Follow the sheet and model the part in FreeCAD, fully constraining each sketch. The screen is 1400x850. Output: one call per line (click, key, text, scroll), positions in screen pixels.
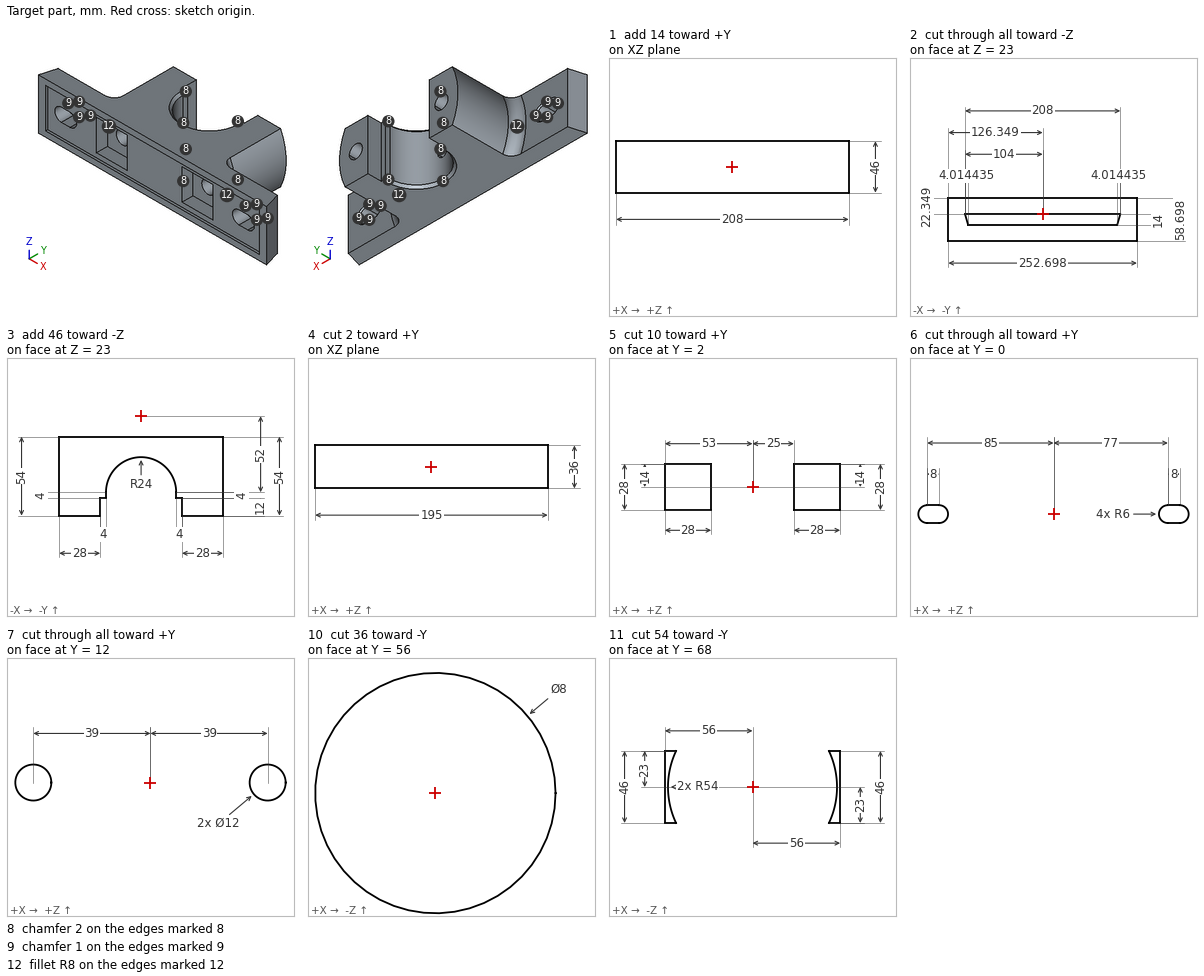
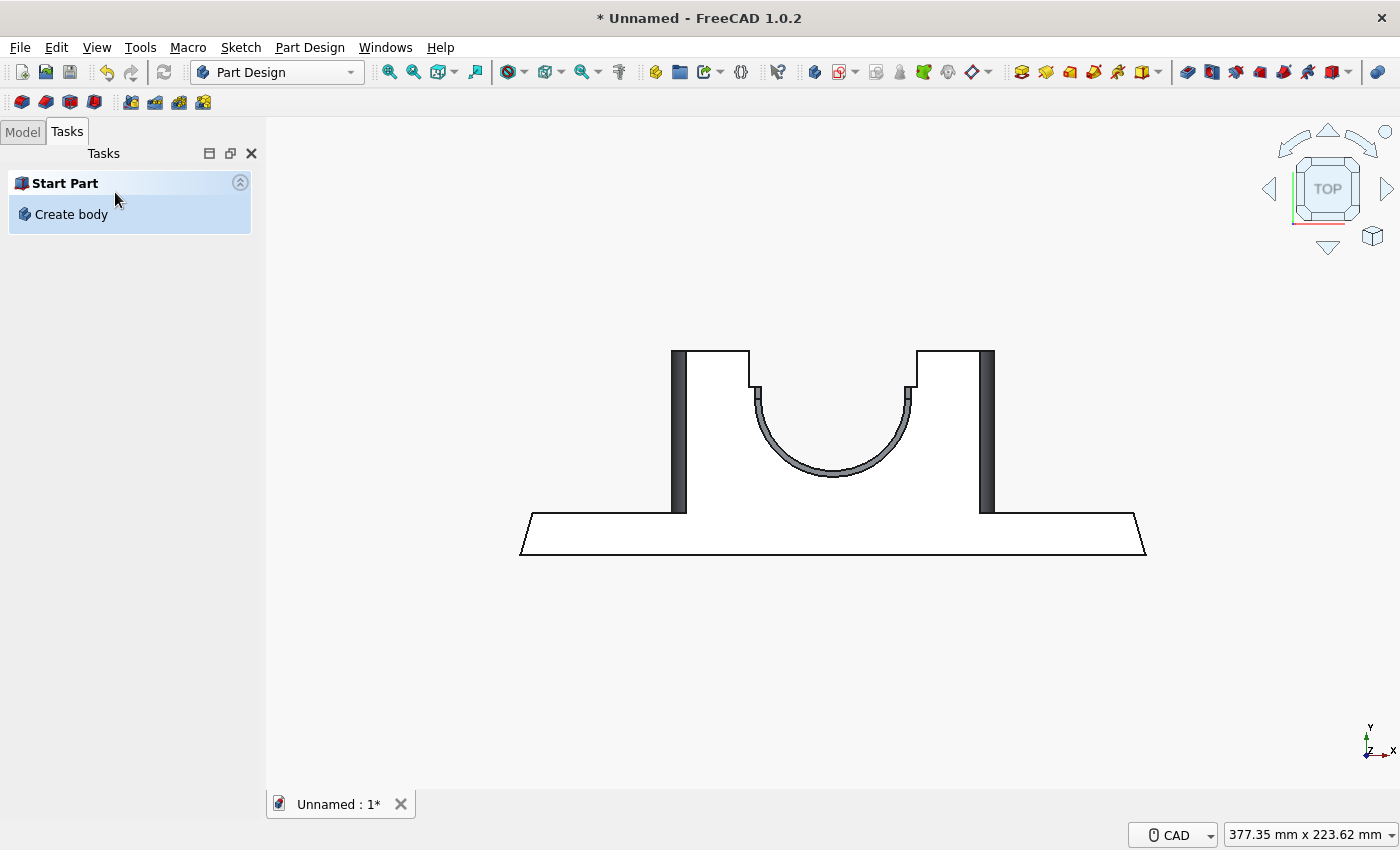
key(1)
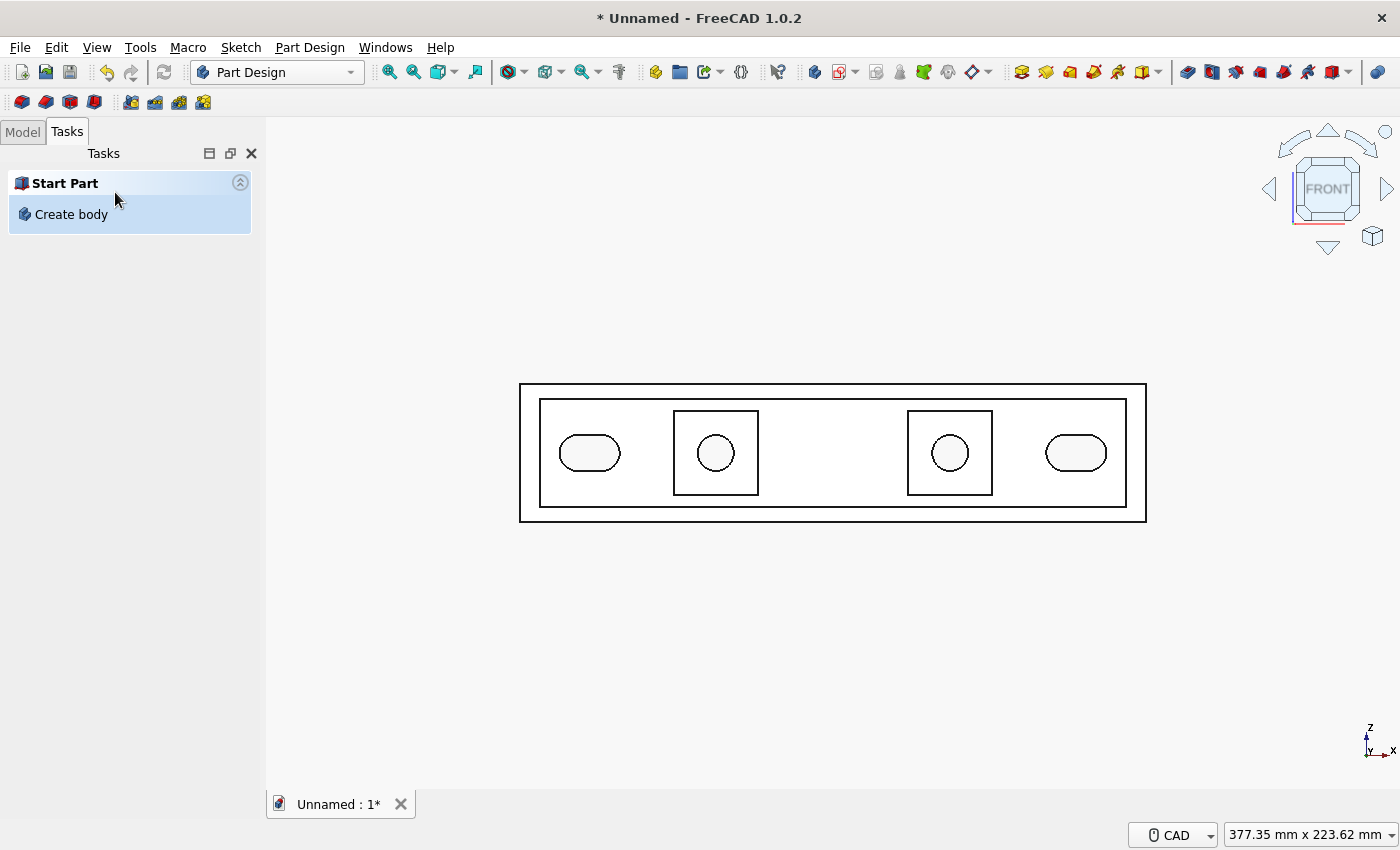
key(3)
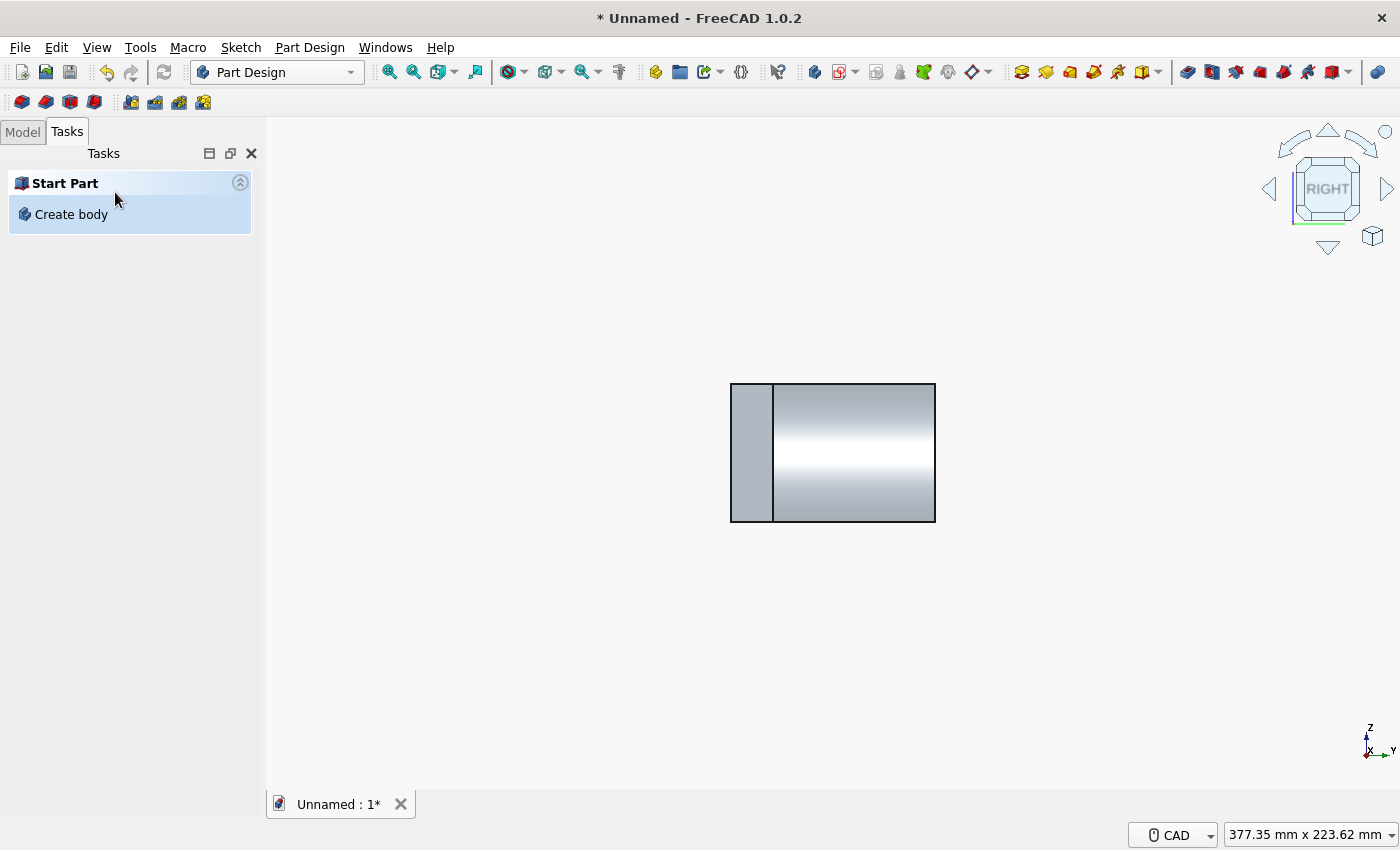
key(v)
key(f)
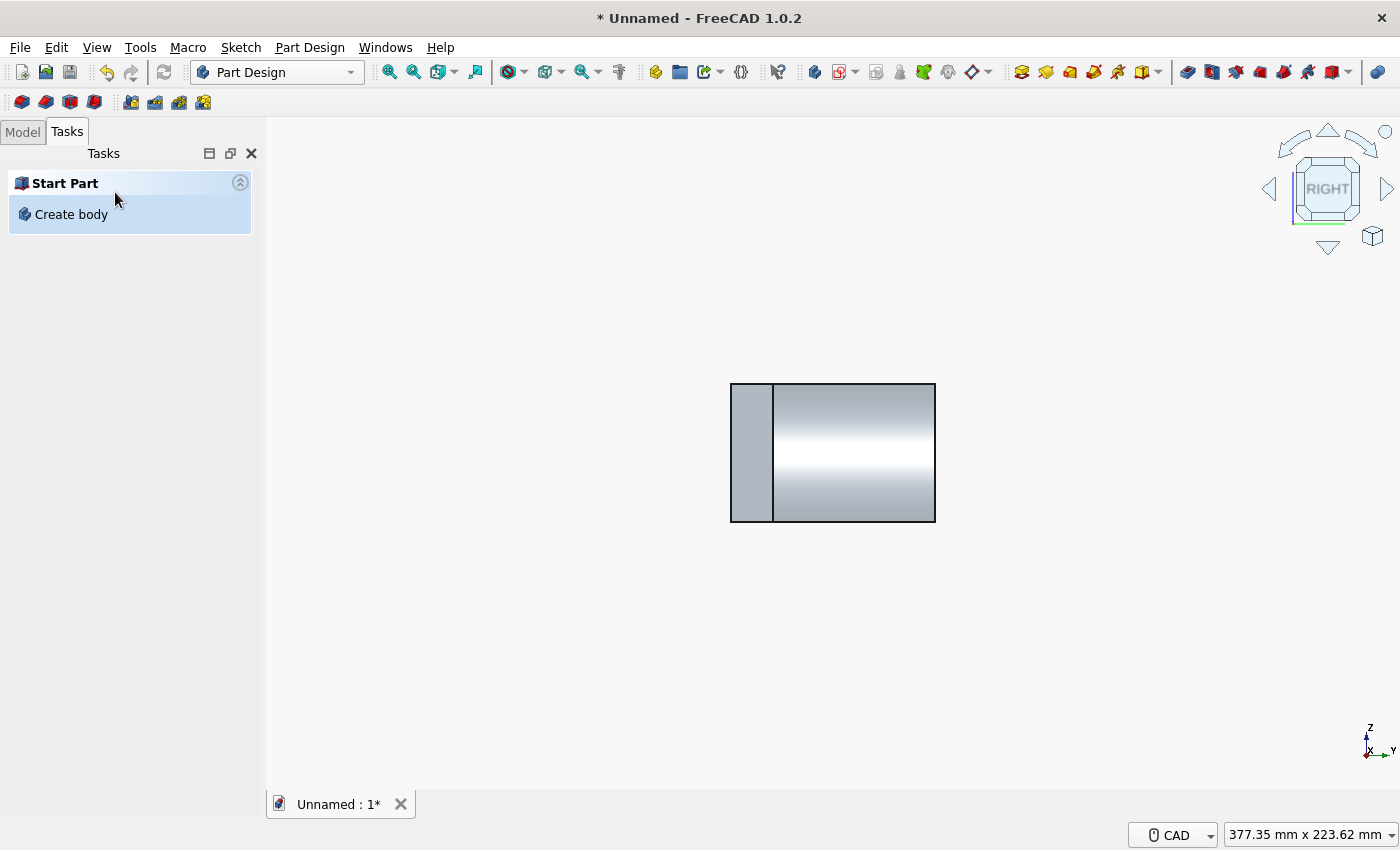
key(5)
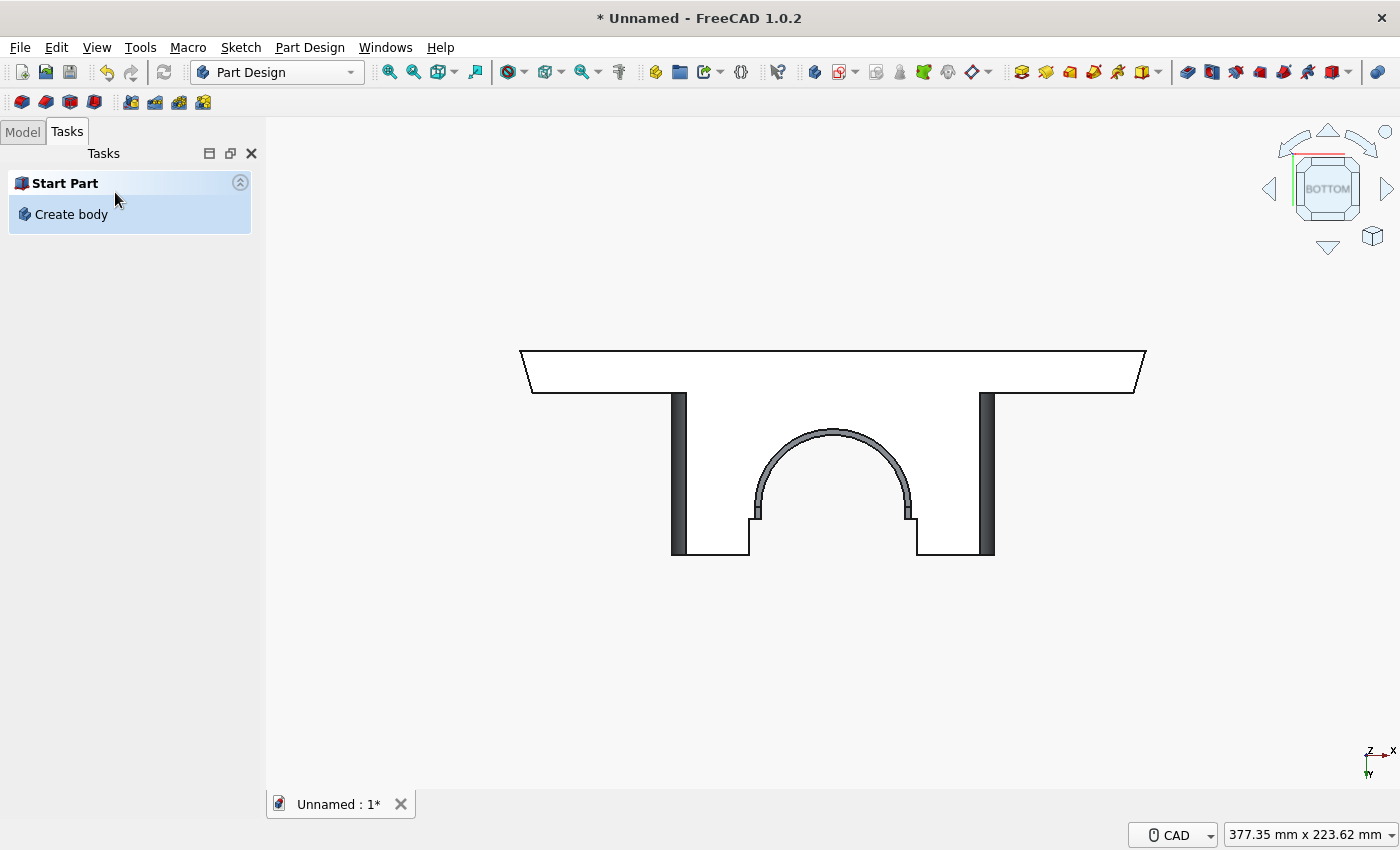
key(4)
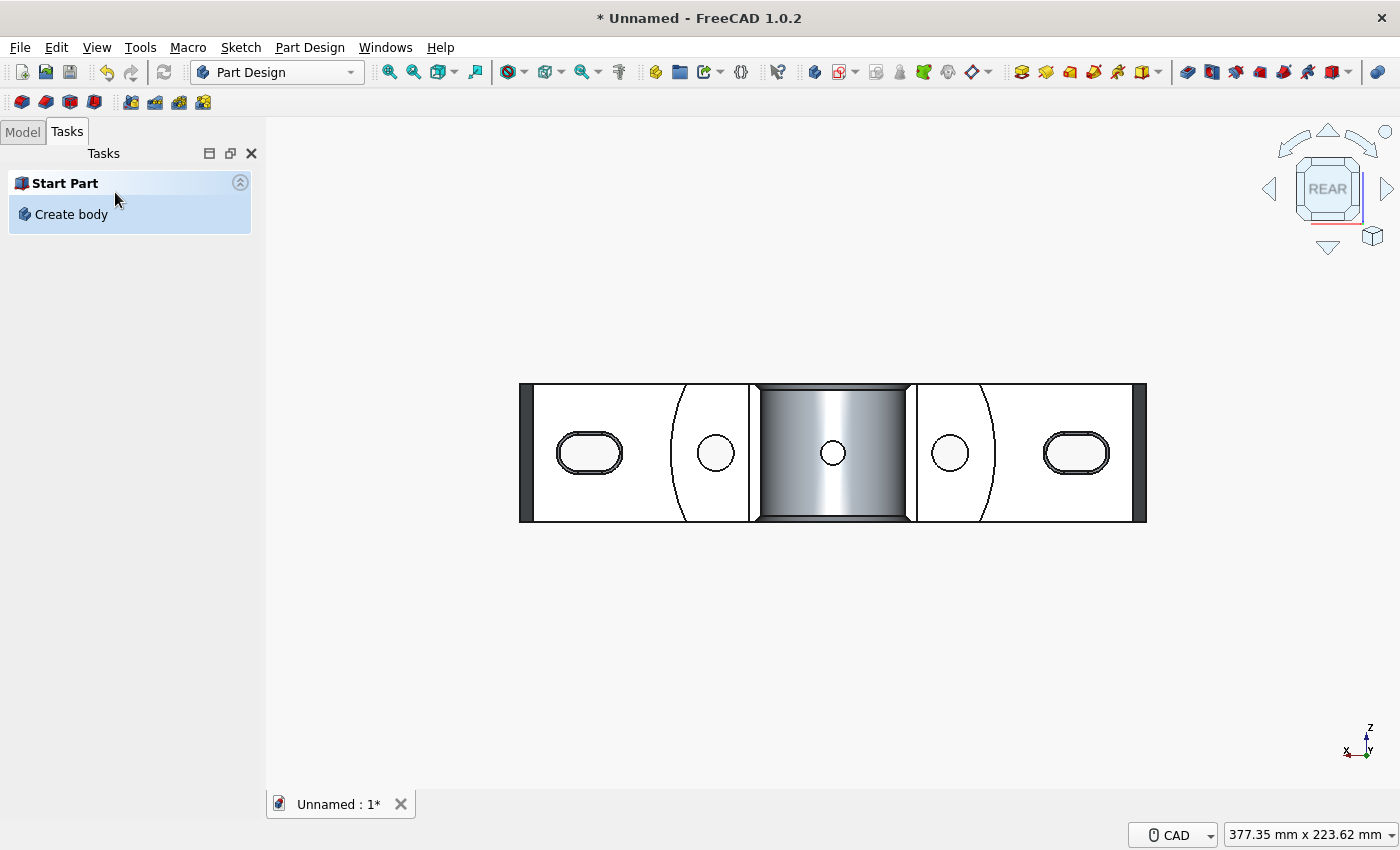
key(6)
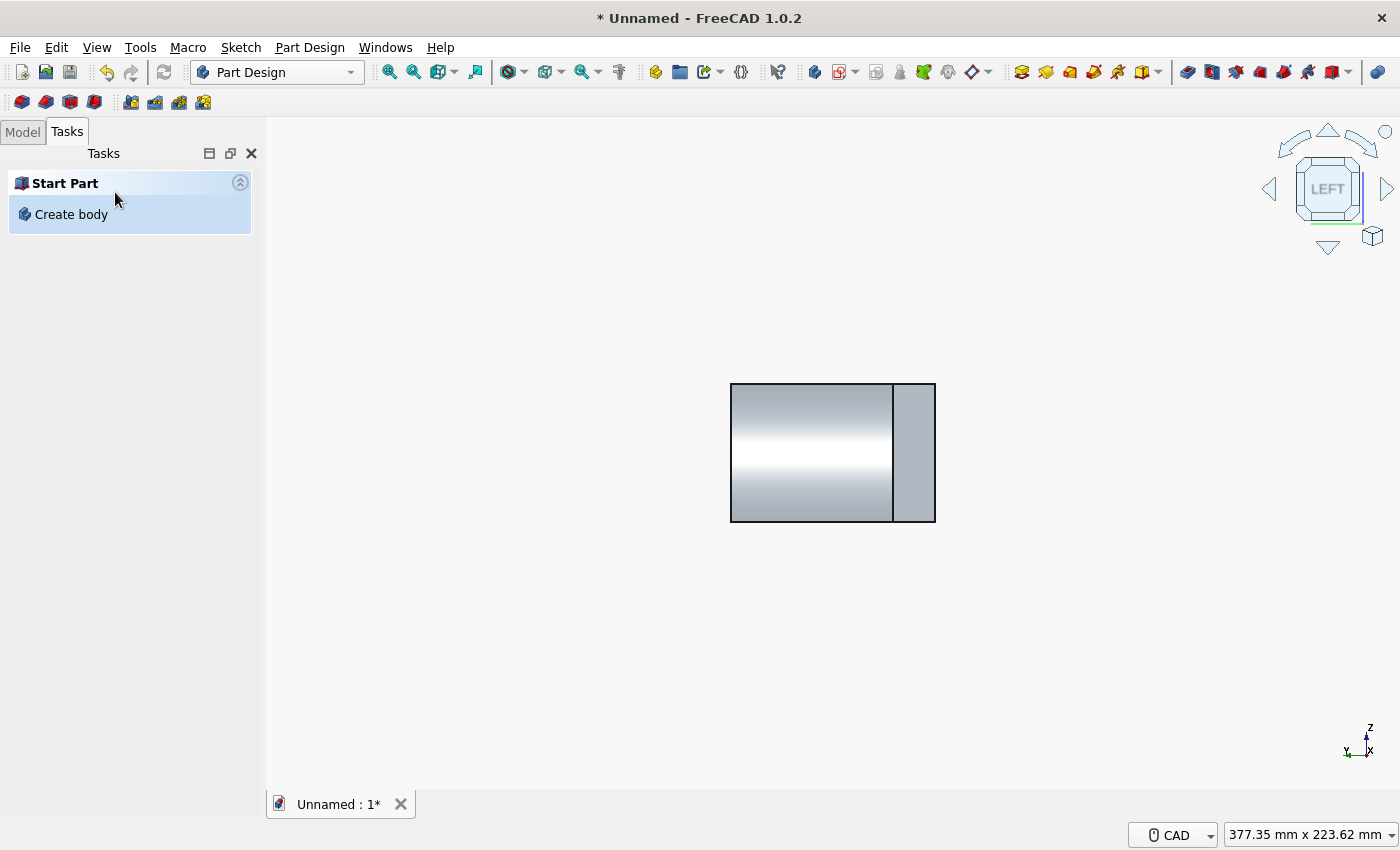
key(v)
key(f)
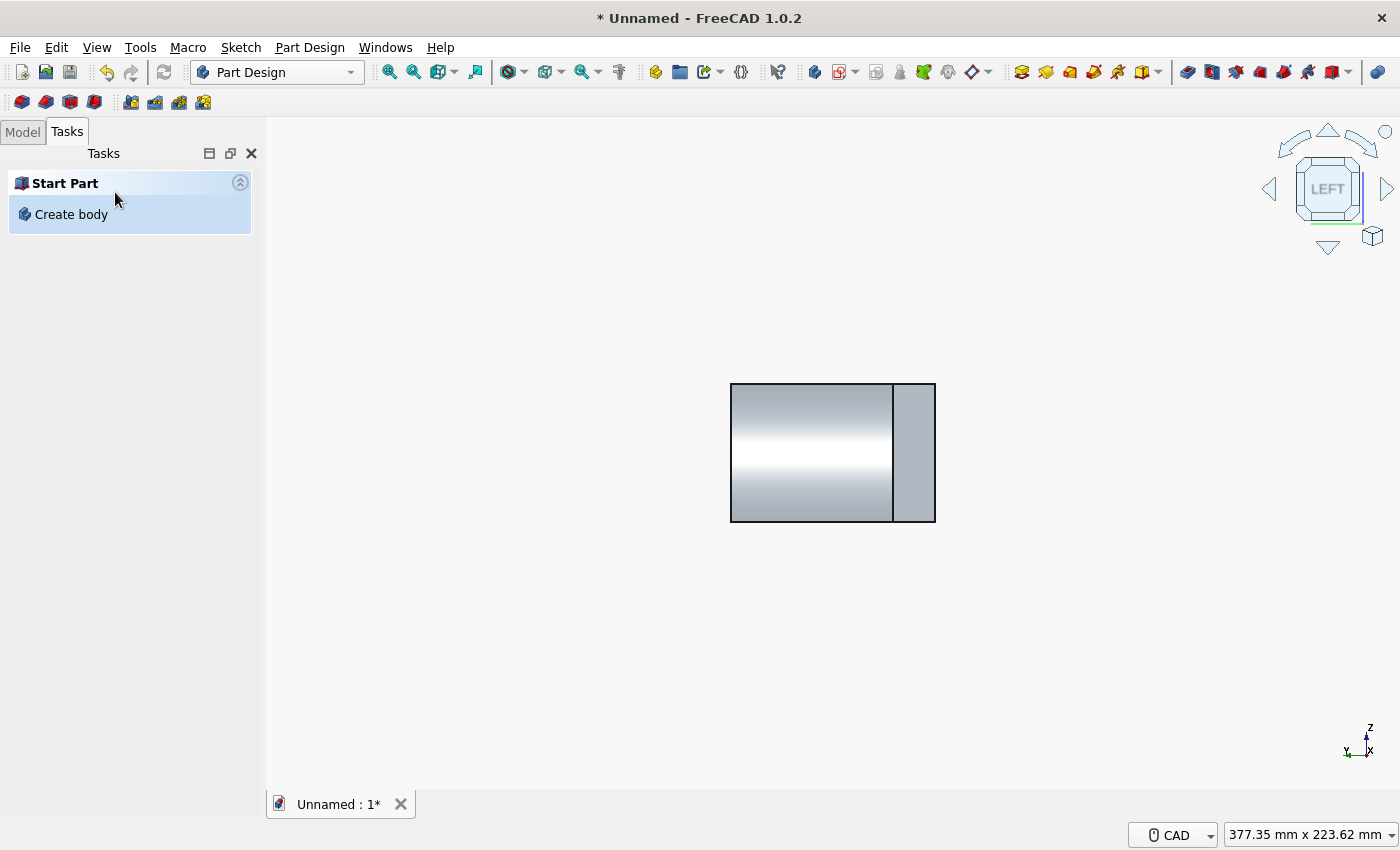
key(v)
key(3)